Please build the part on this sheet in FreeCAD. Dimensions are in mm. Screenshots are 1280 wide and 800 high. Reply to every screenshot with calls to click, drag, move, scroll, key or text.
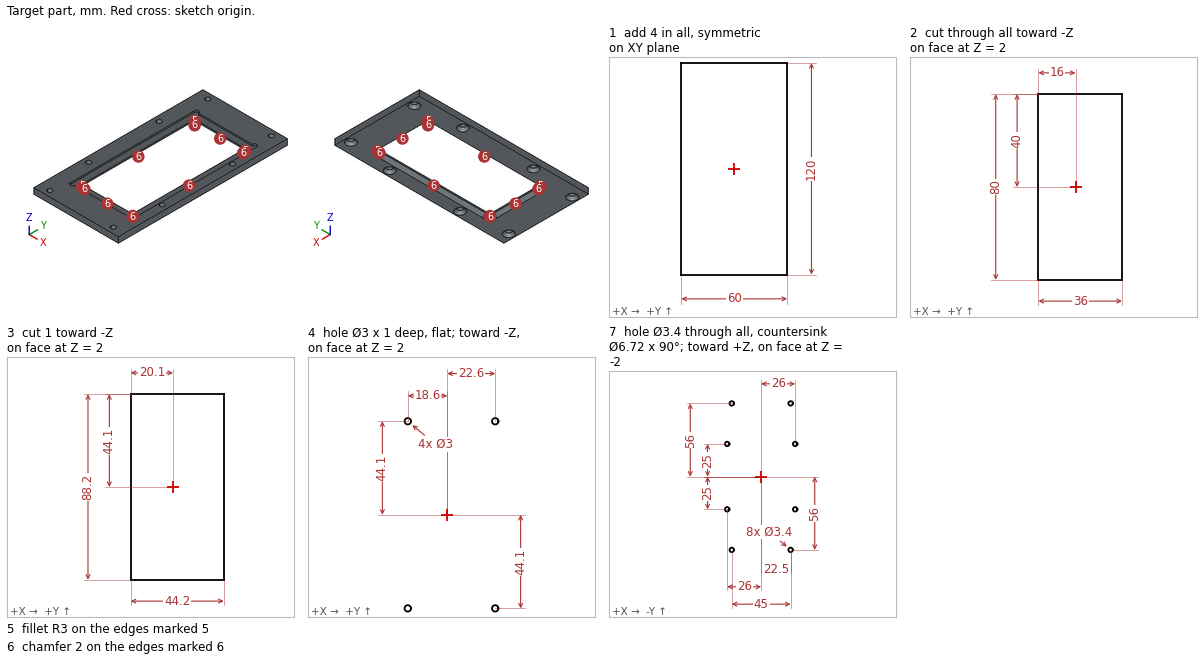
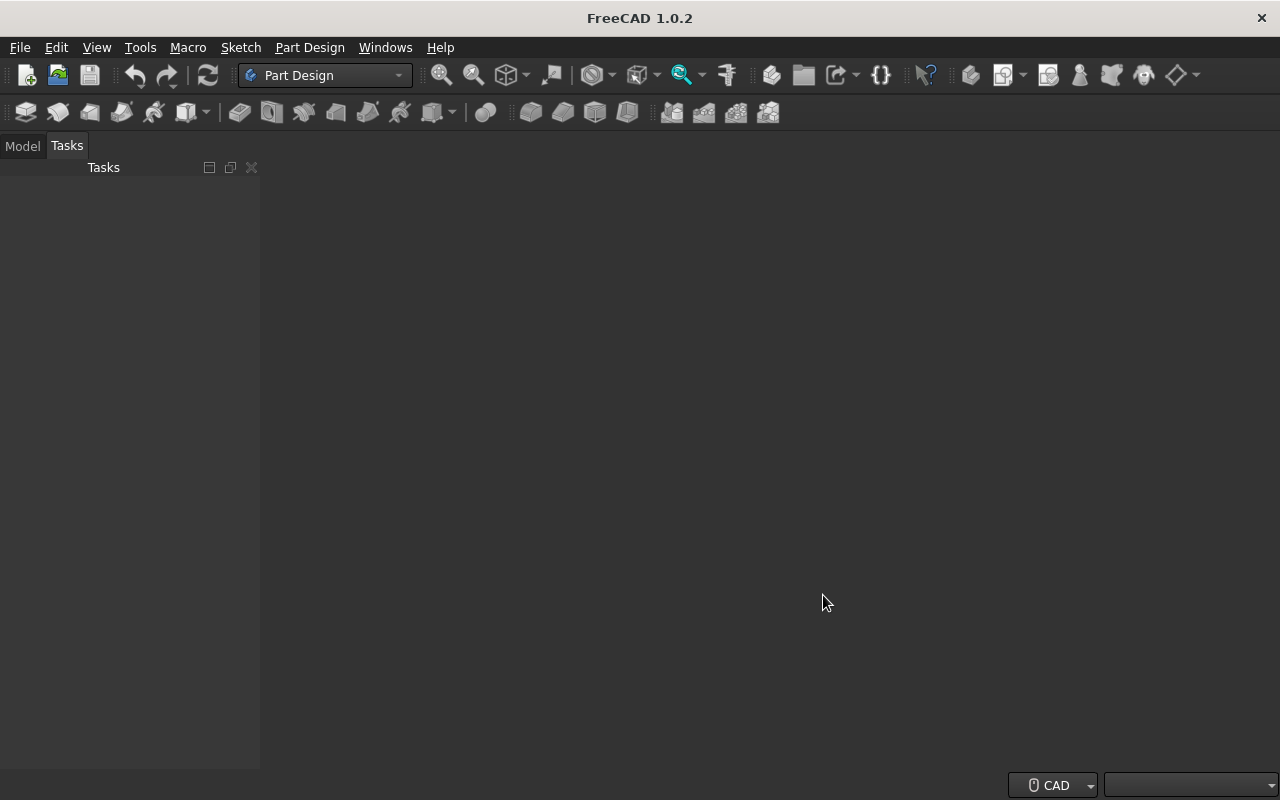
click(26, 76)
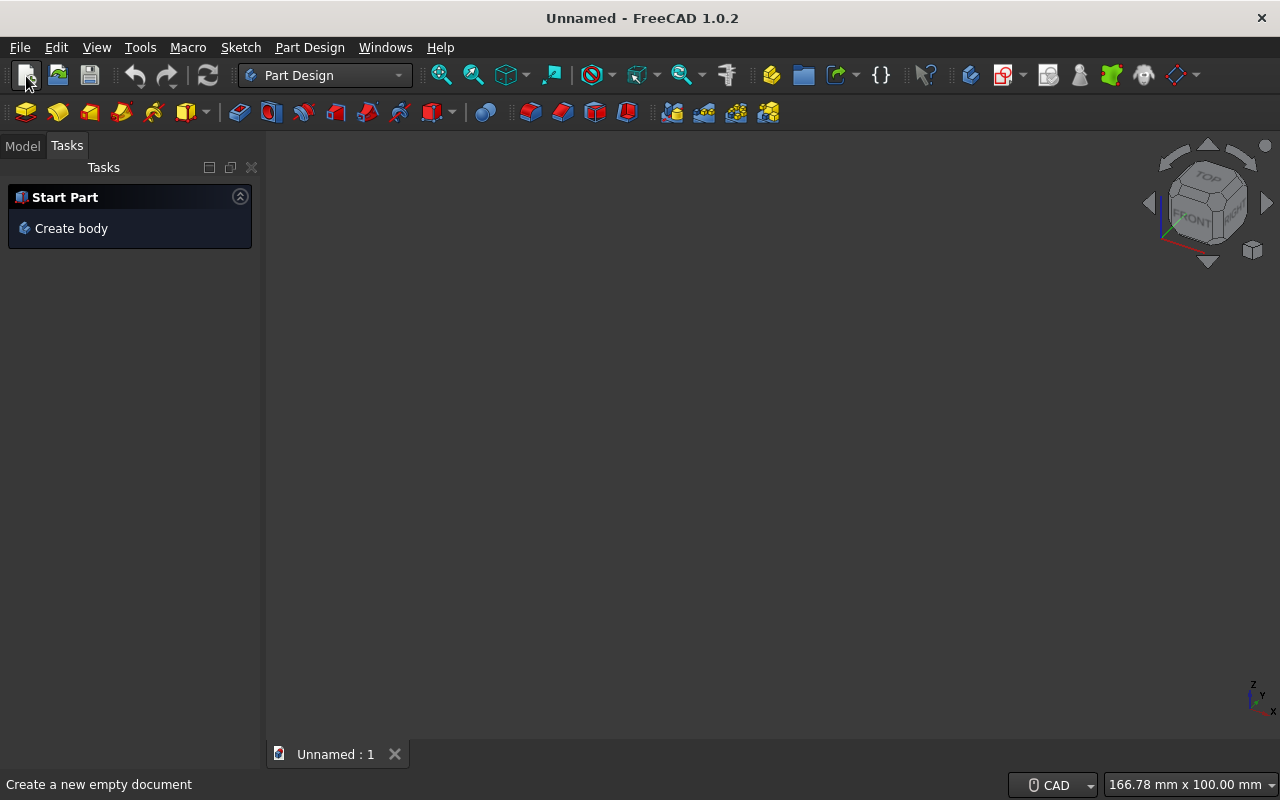
click(1004, 76)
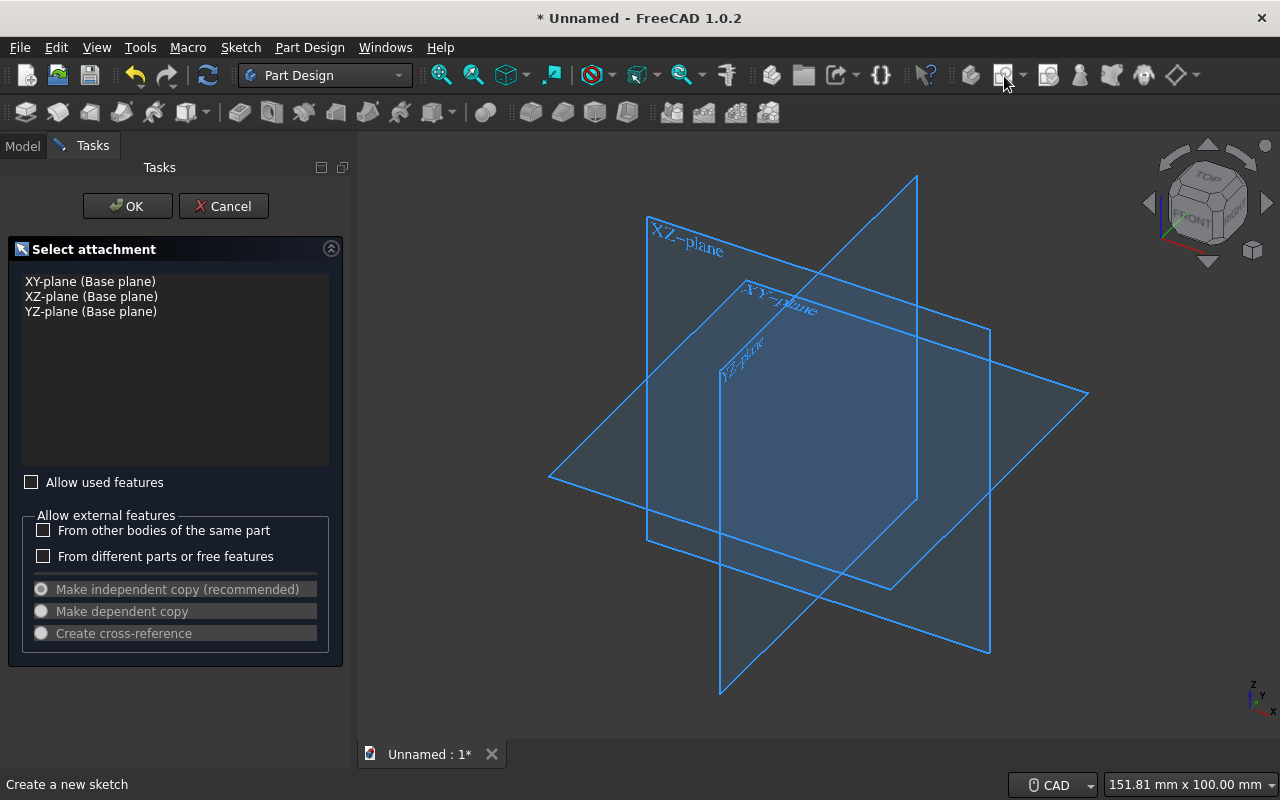
click(82, 282)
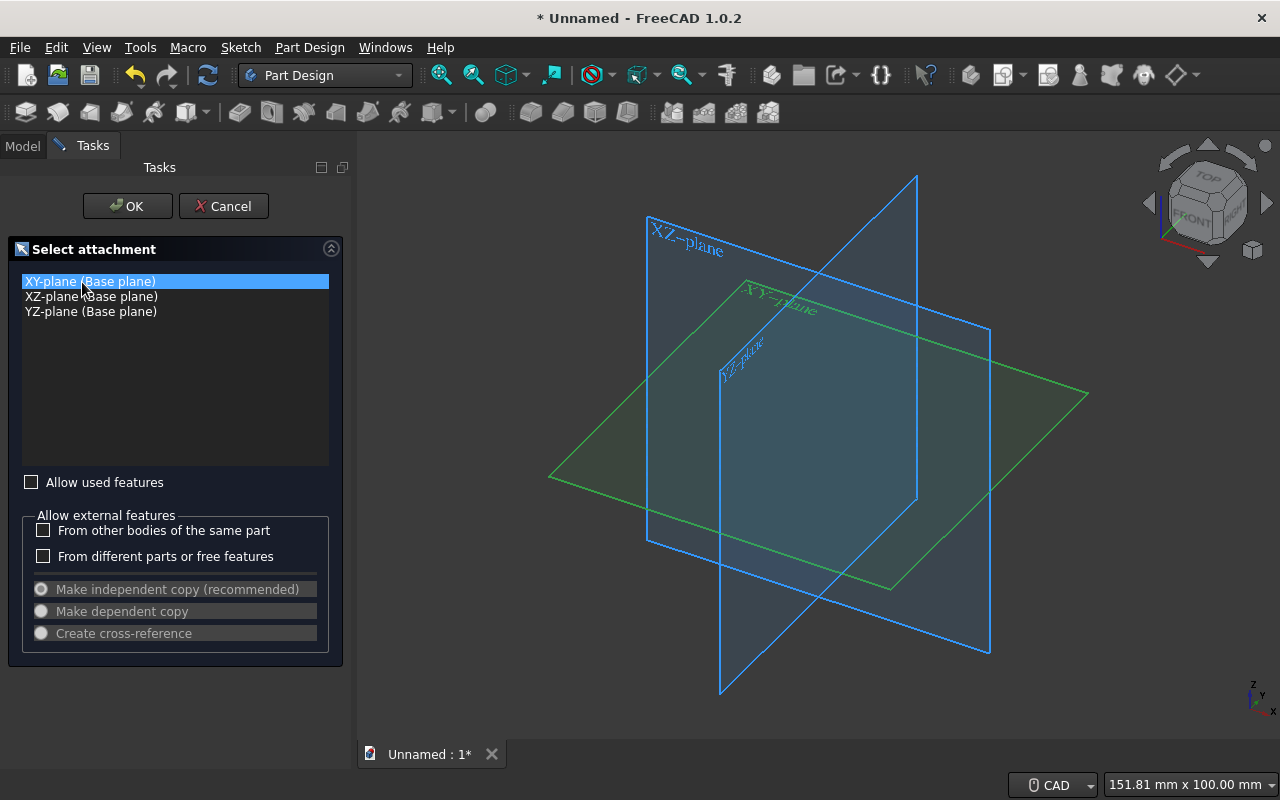
click(128, 206)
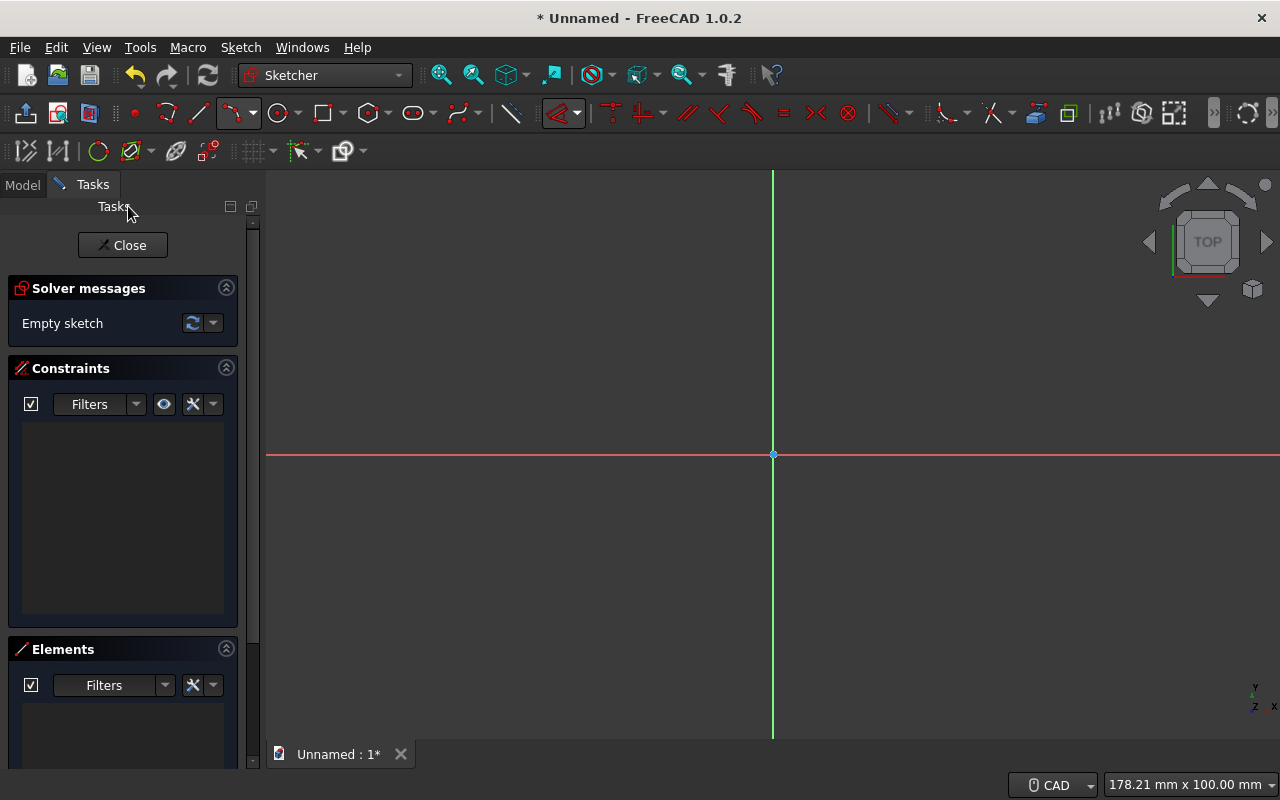
scroll(621, 454, down, 3)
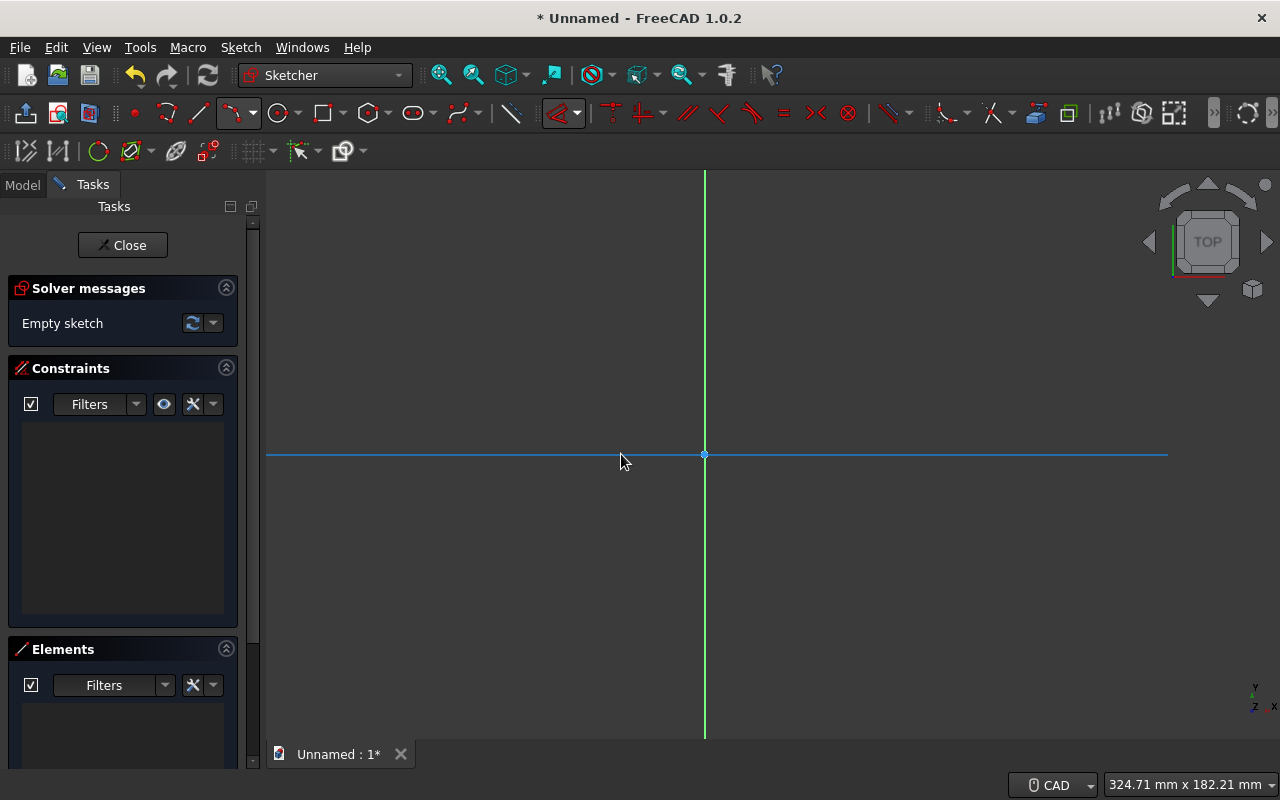
key(g)
key(v)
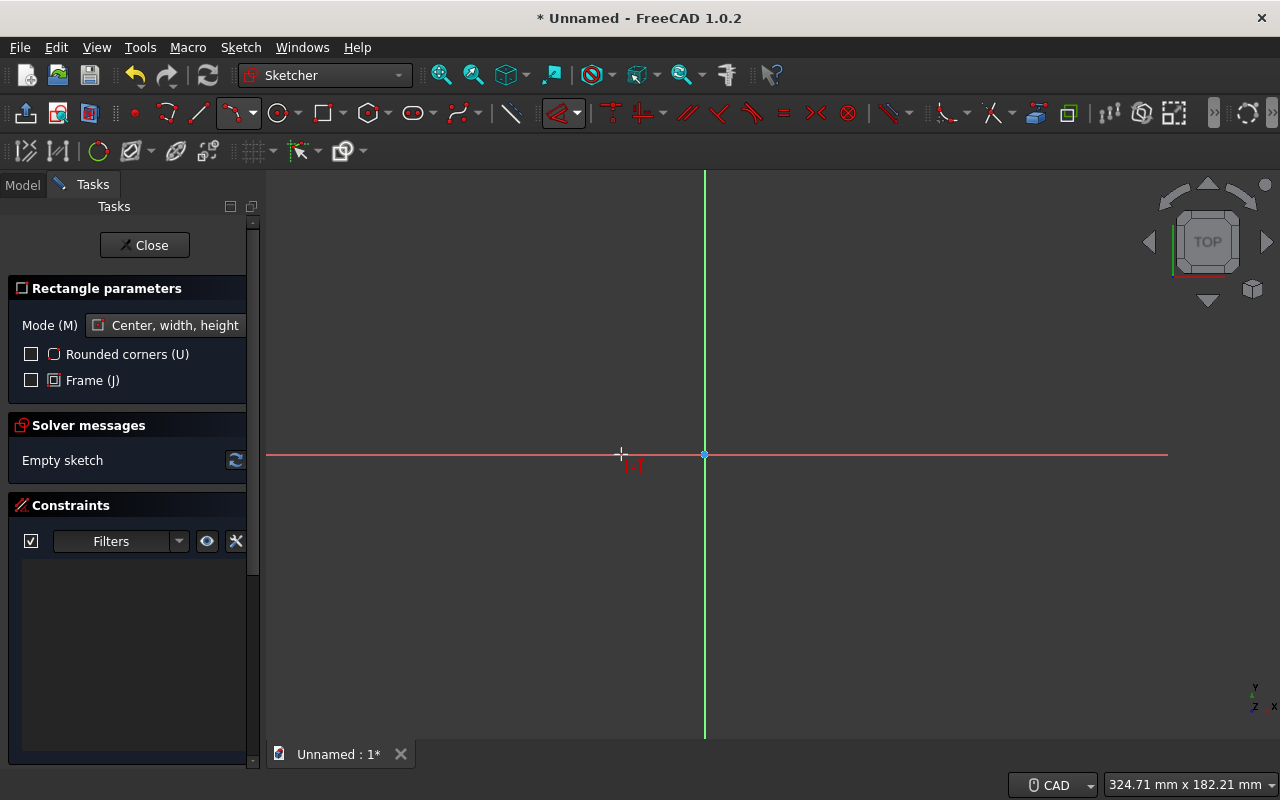
click(705, 454)
click(798, 267)
key(Escape)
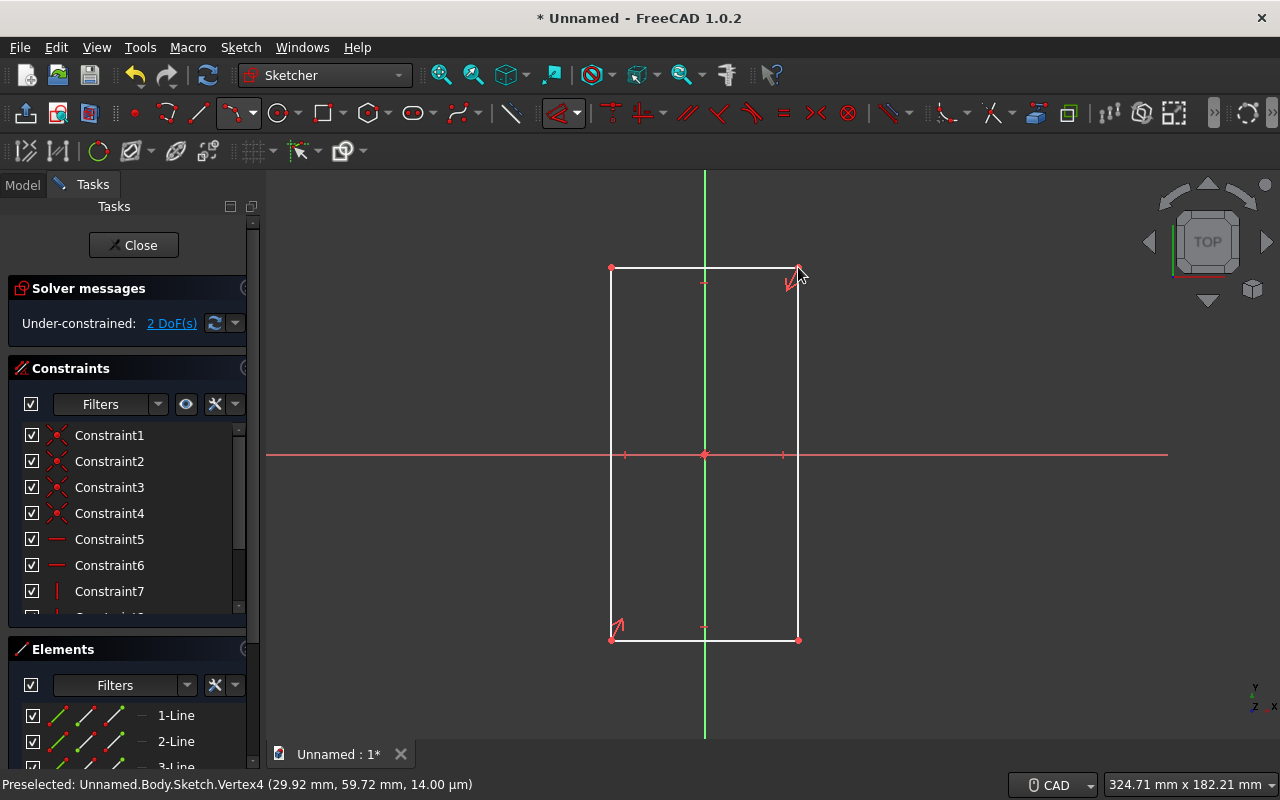
click(558, 114)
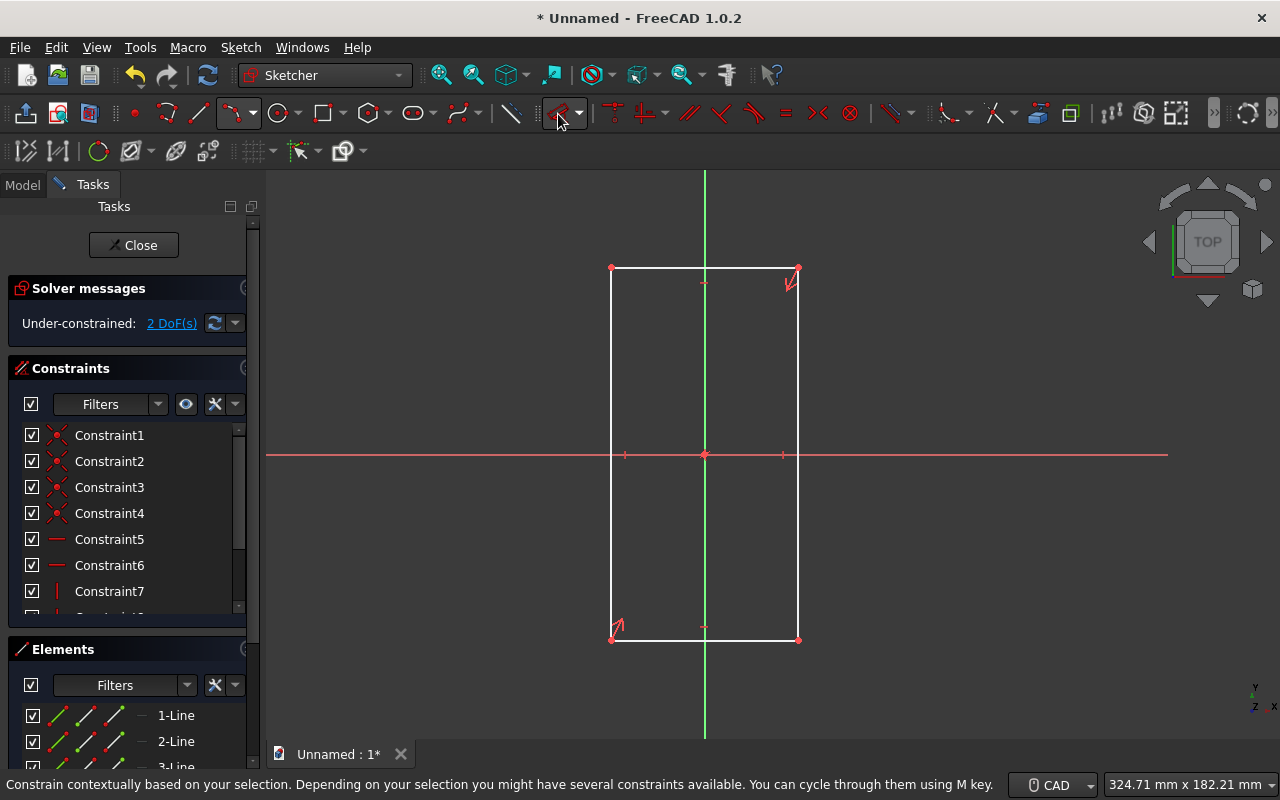
click(667, 641)
click(662, 675)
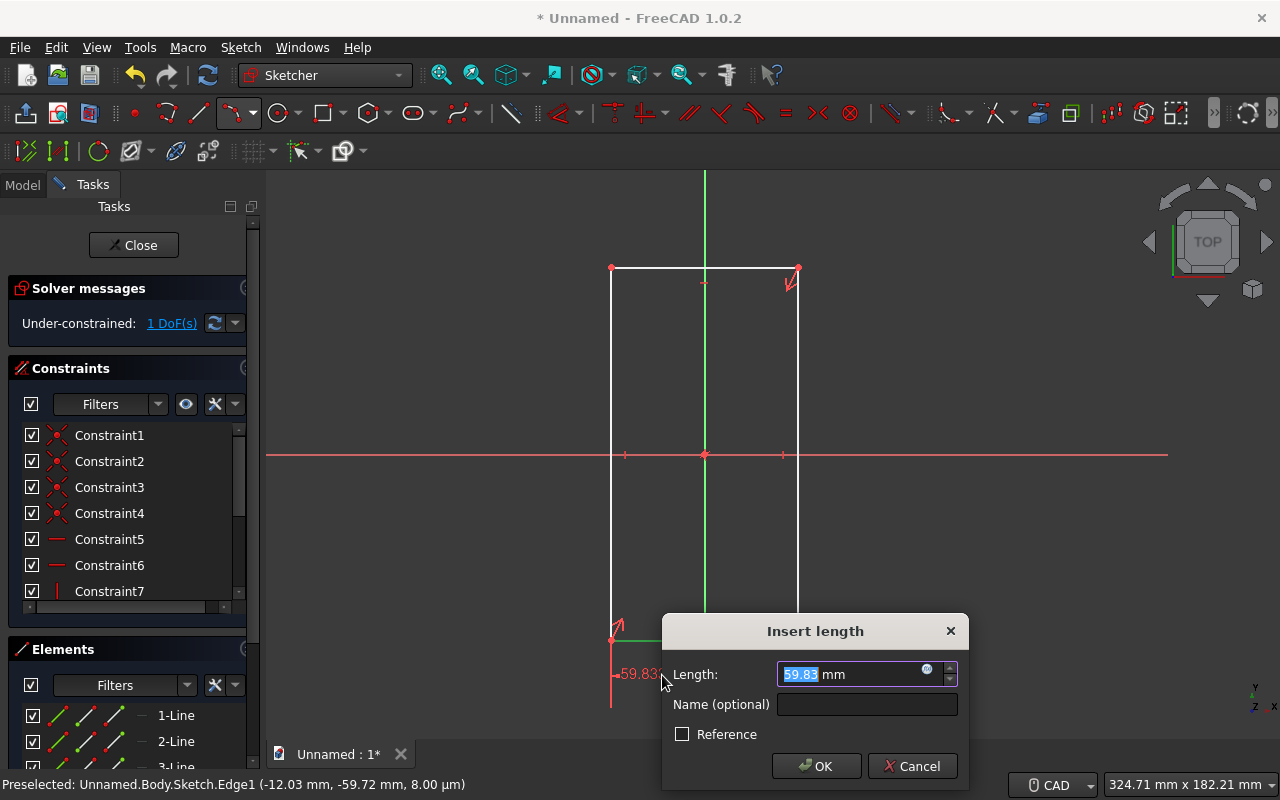
text(60)
key(Return)